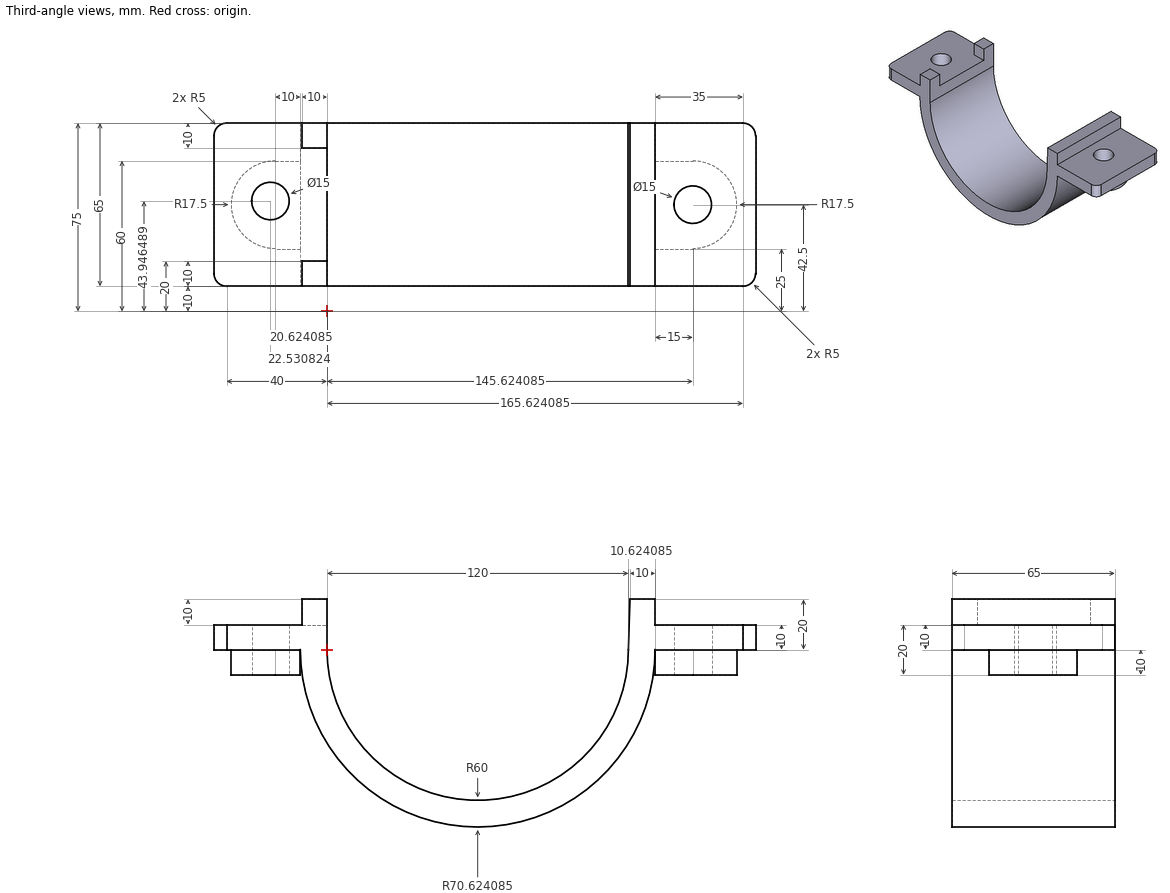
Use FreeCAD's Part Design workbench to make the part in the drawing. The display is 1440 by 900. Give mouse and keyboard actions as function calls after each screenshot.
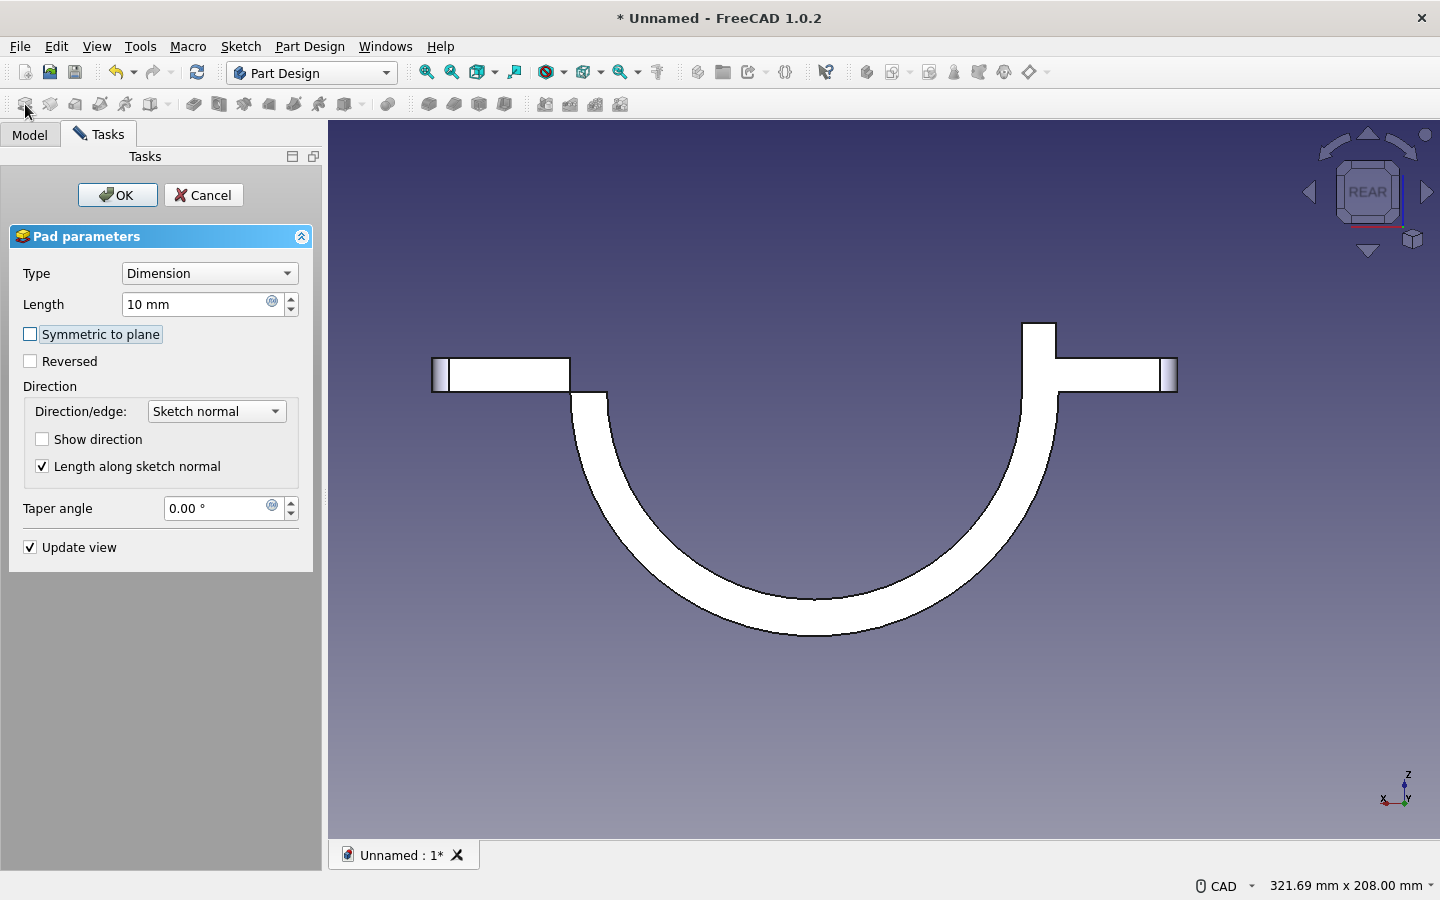
click(118, 195)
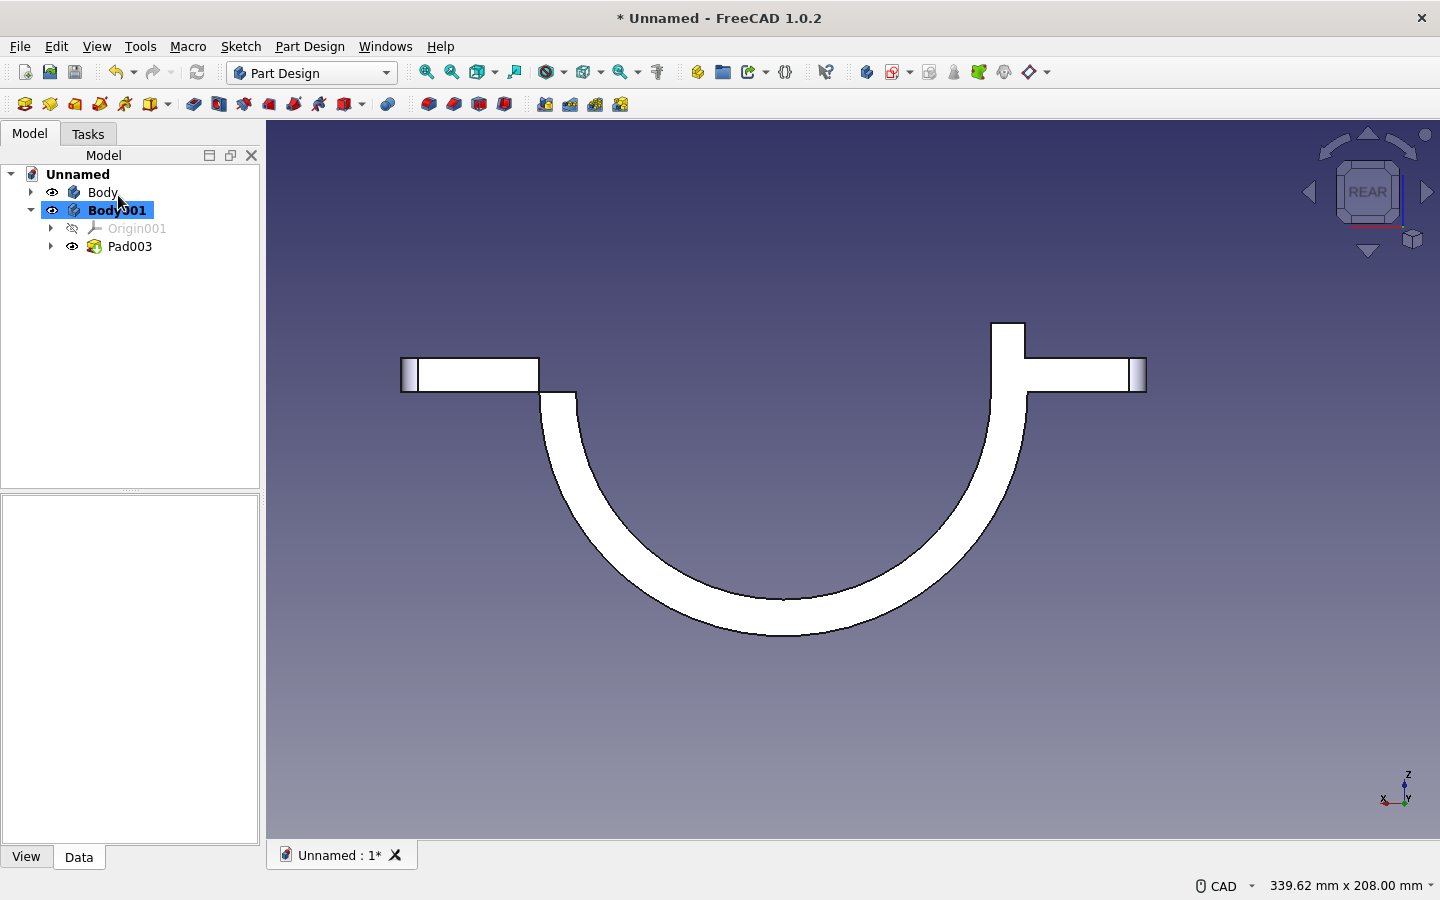
click(427, 72)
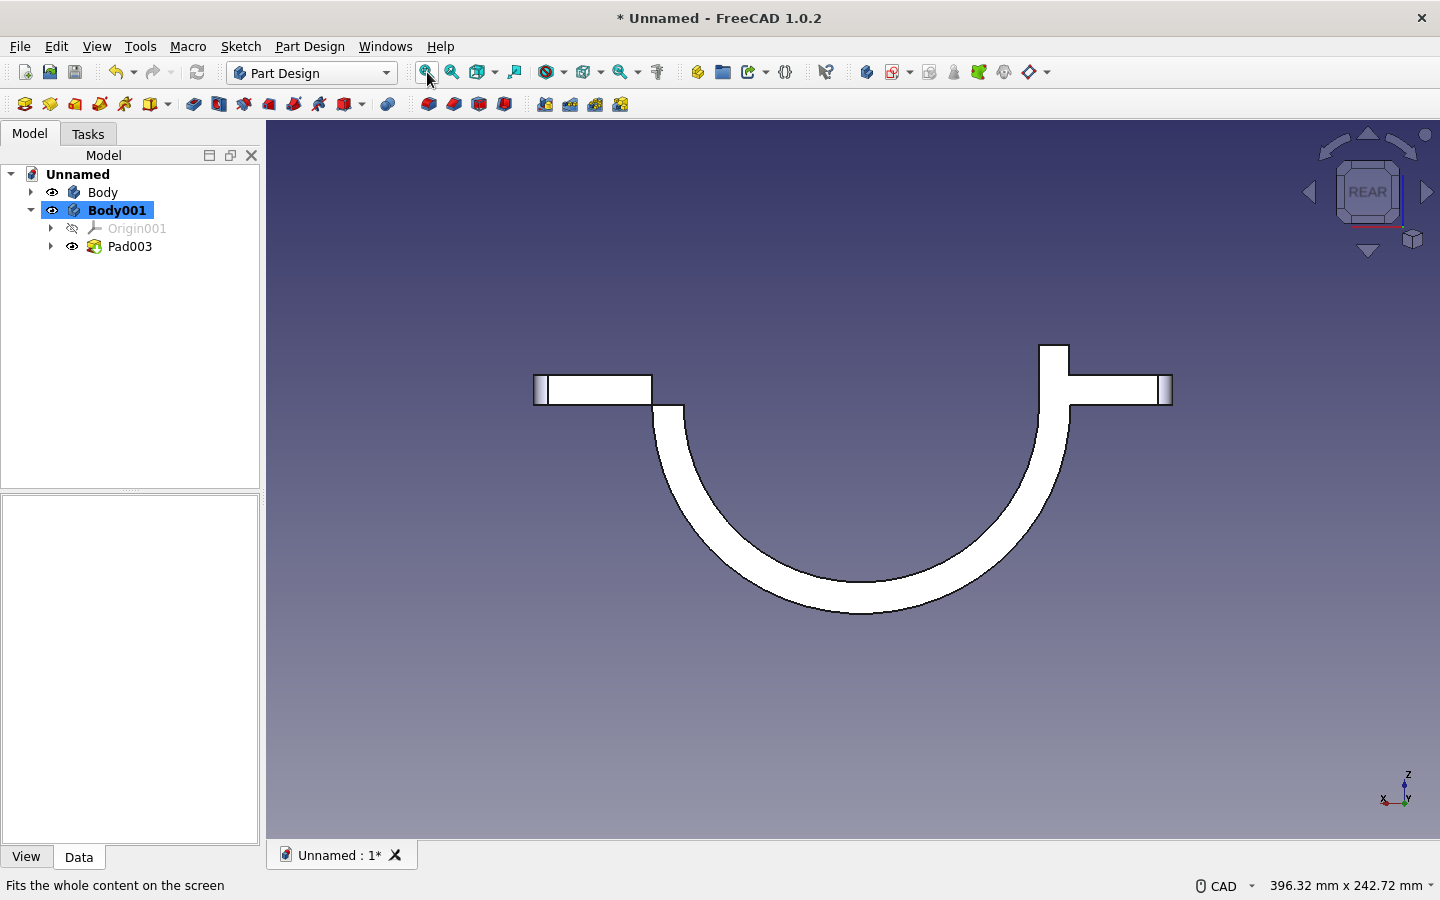
double_click(97, 192)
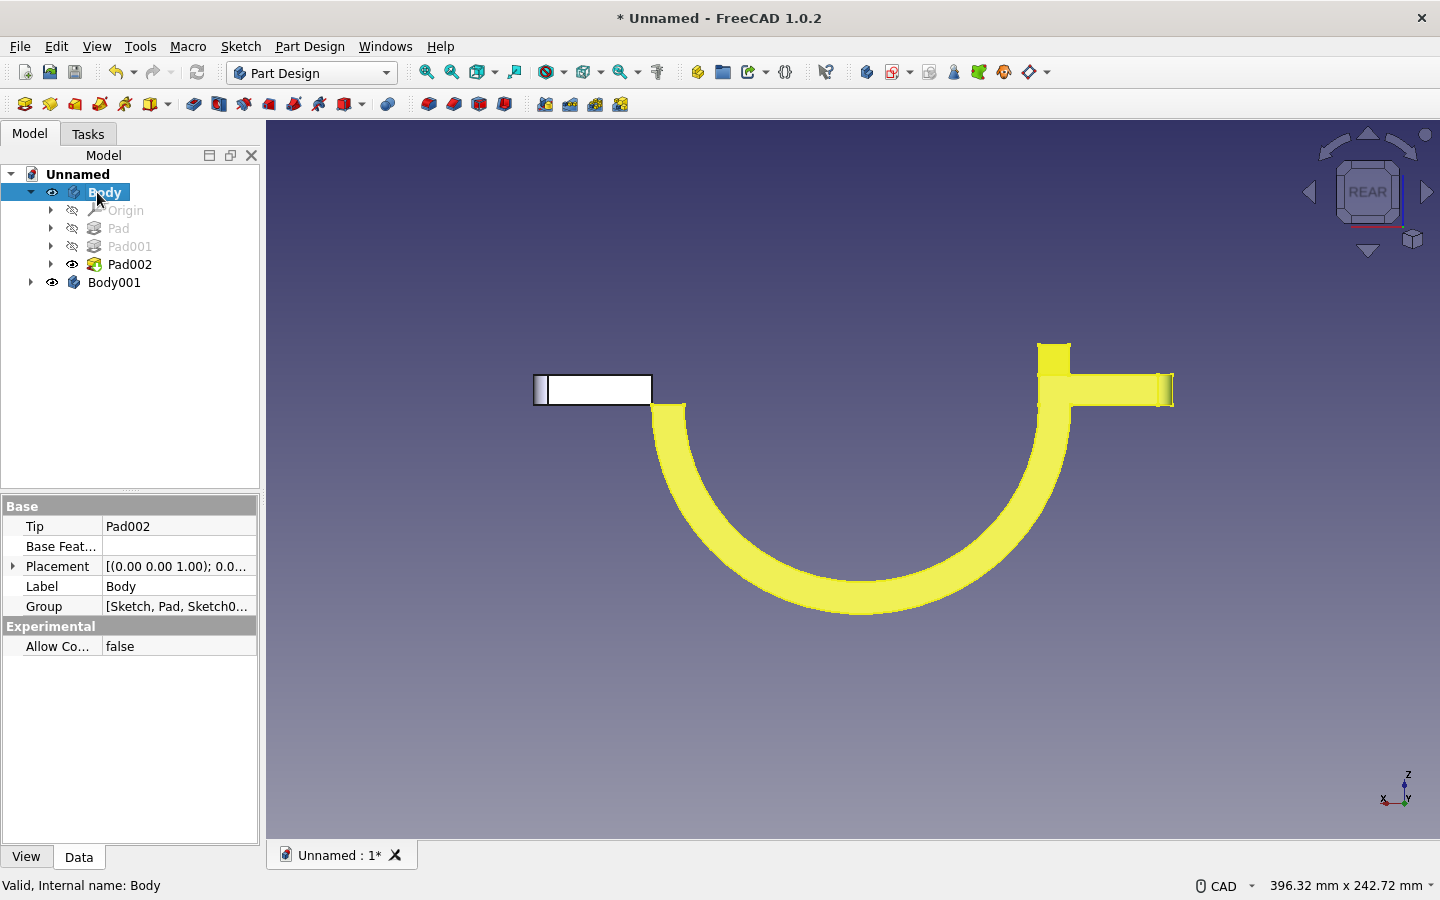
click(97, 192)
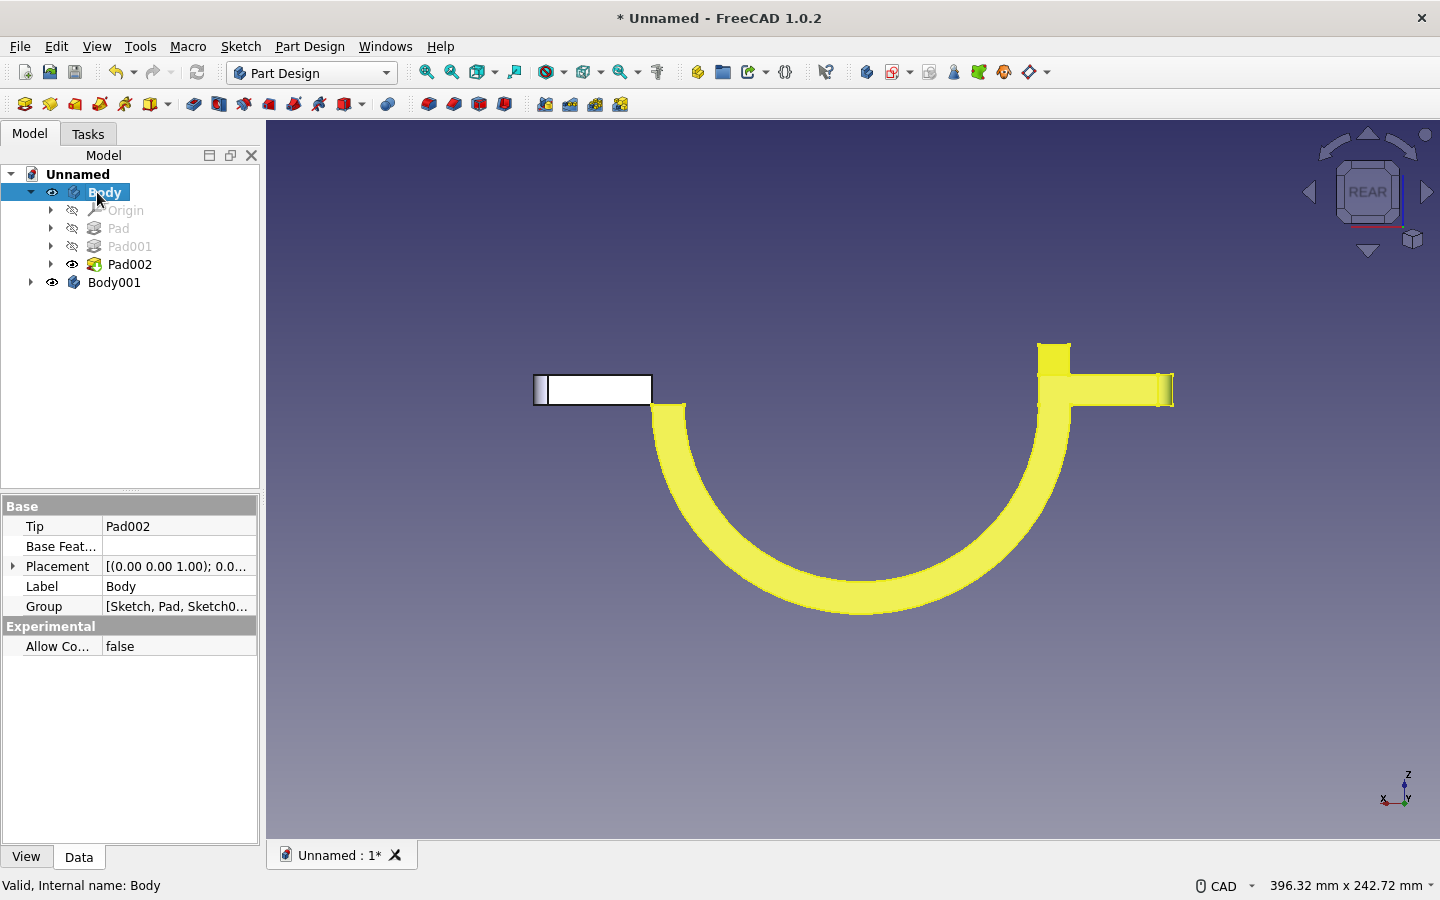
click(148, 646)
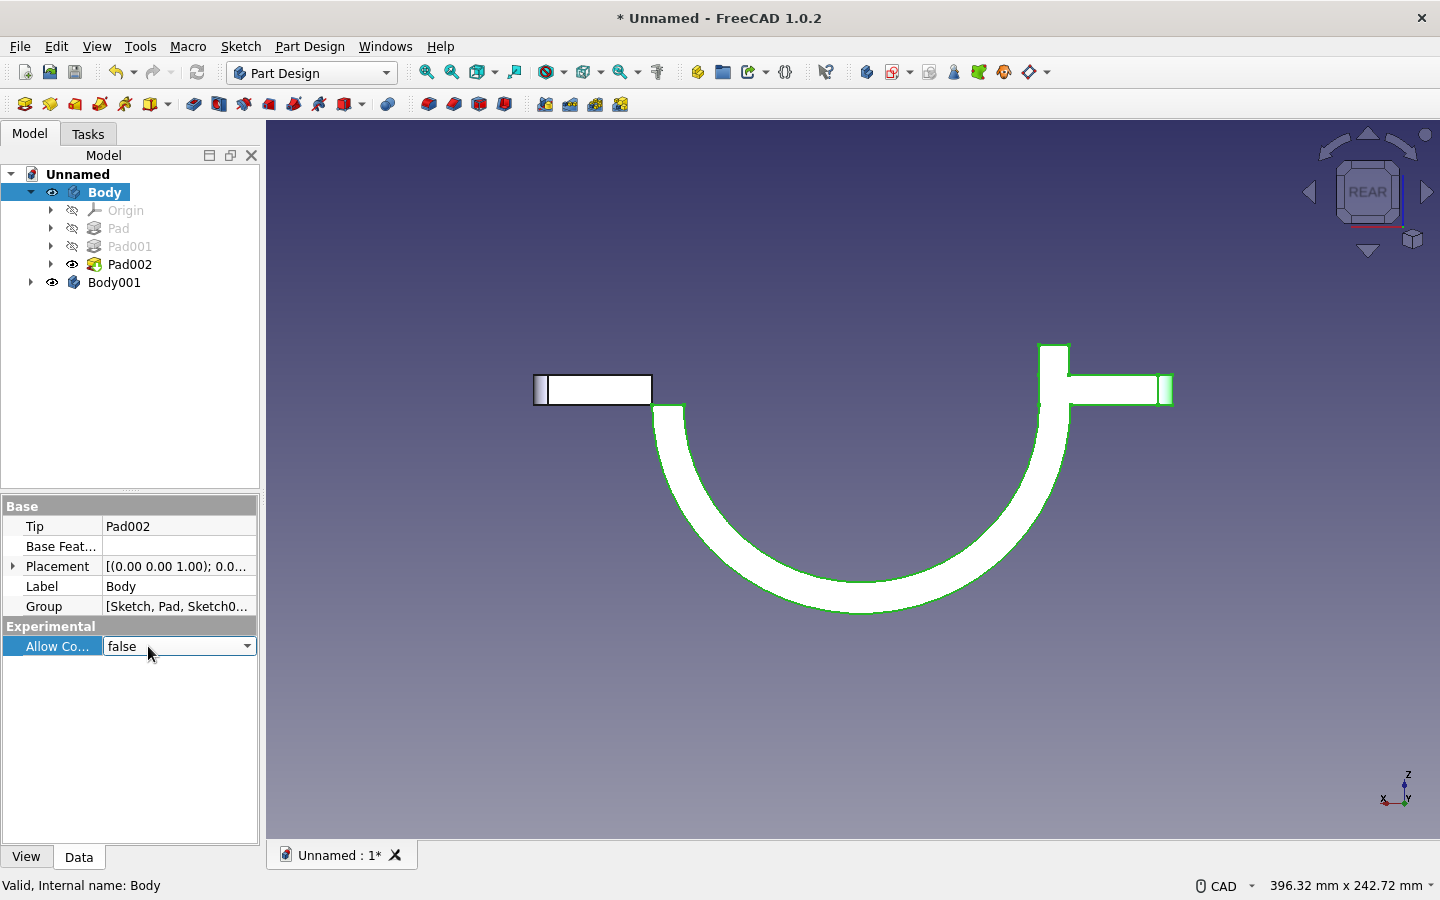
click(148, 646)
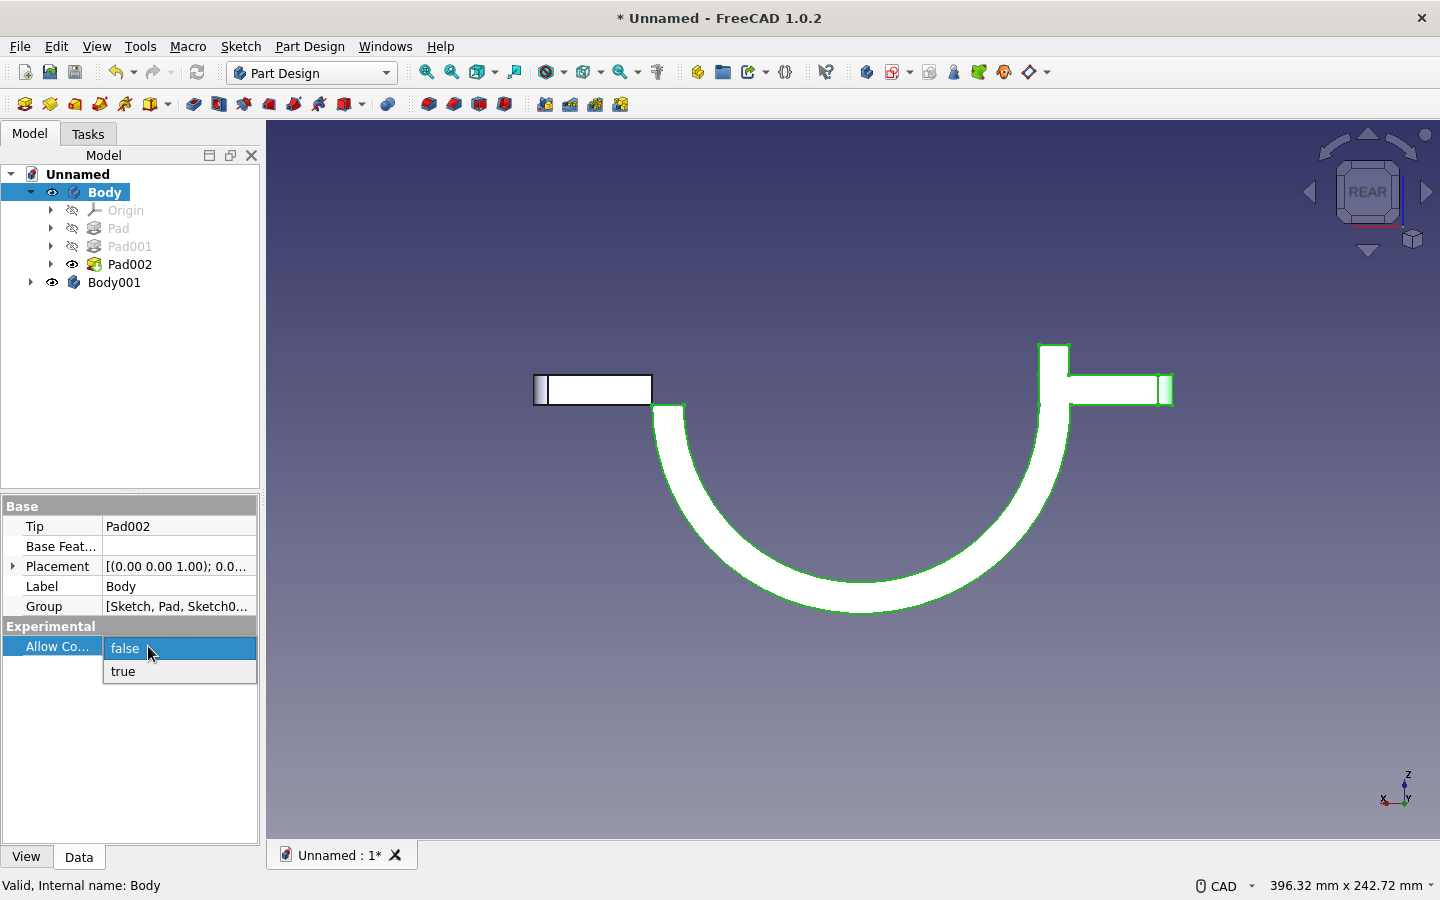
click(178, 672)
key(Return)